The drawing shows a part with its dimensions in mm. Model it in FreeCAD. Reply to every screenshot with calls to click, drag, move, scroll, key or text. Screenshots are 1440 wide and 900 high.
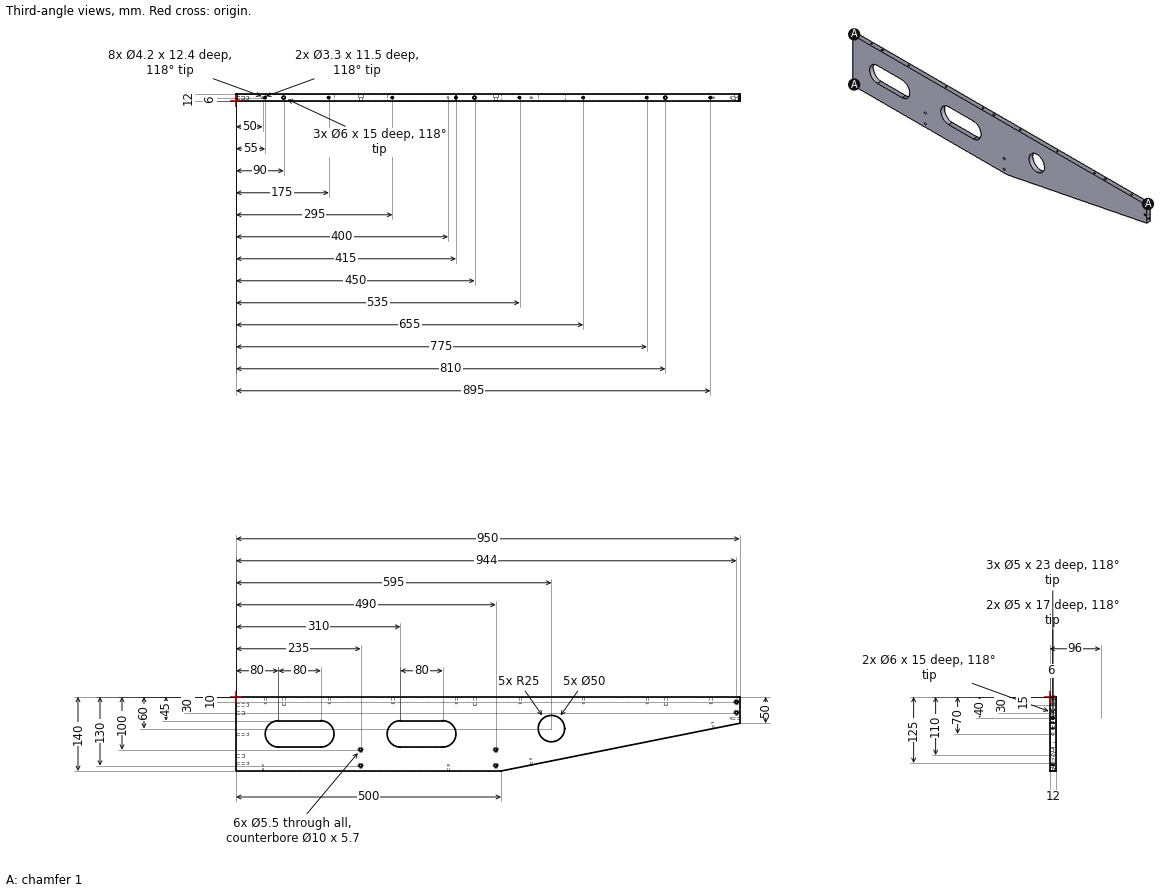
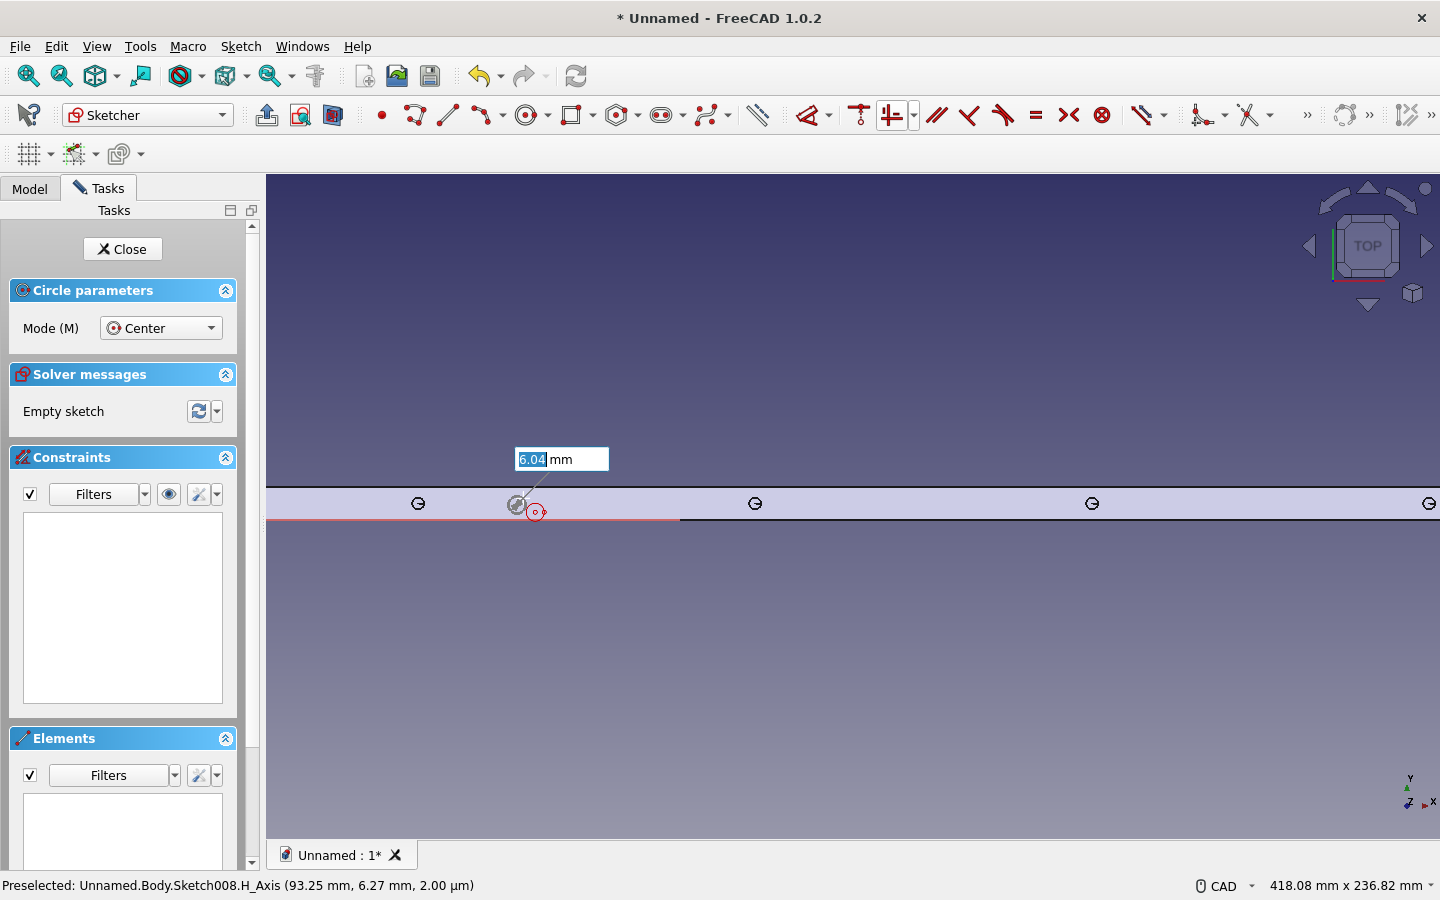
text(6)
key(Return)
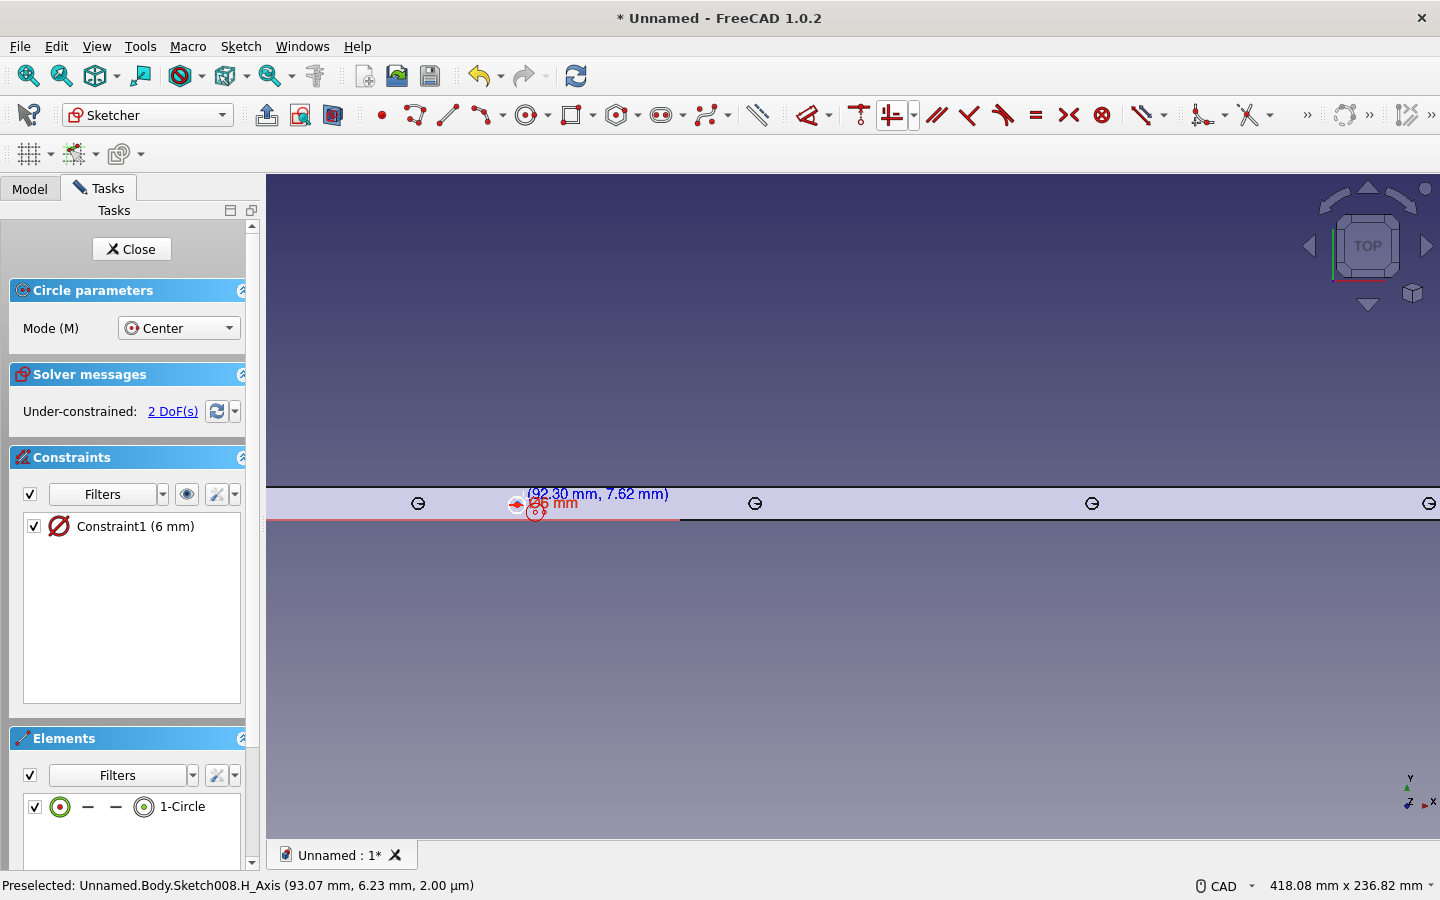
scroll(517, 506, down, 6)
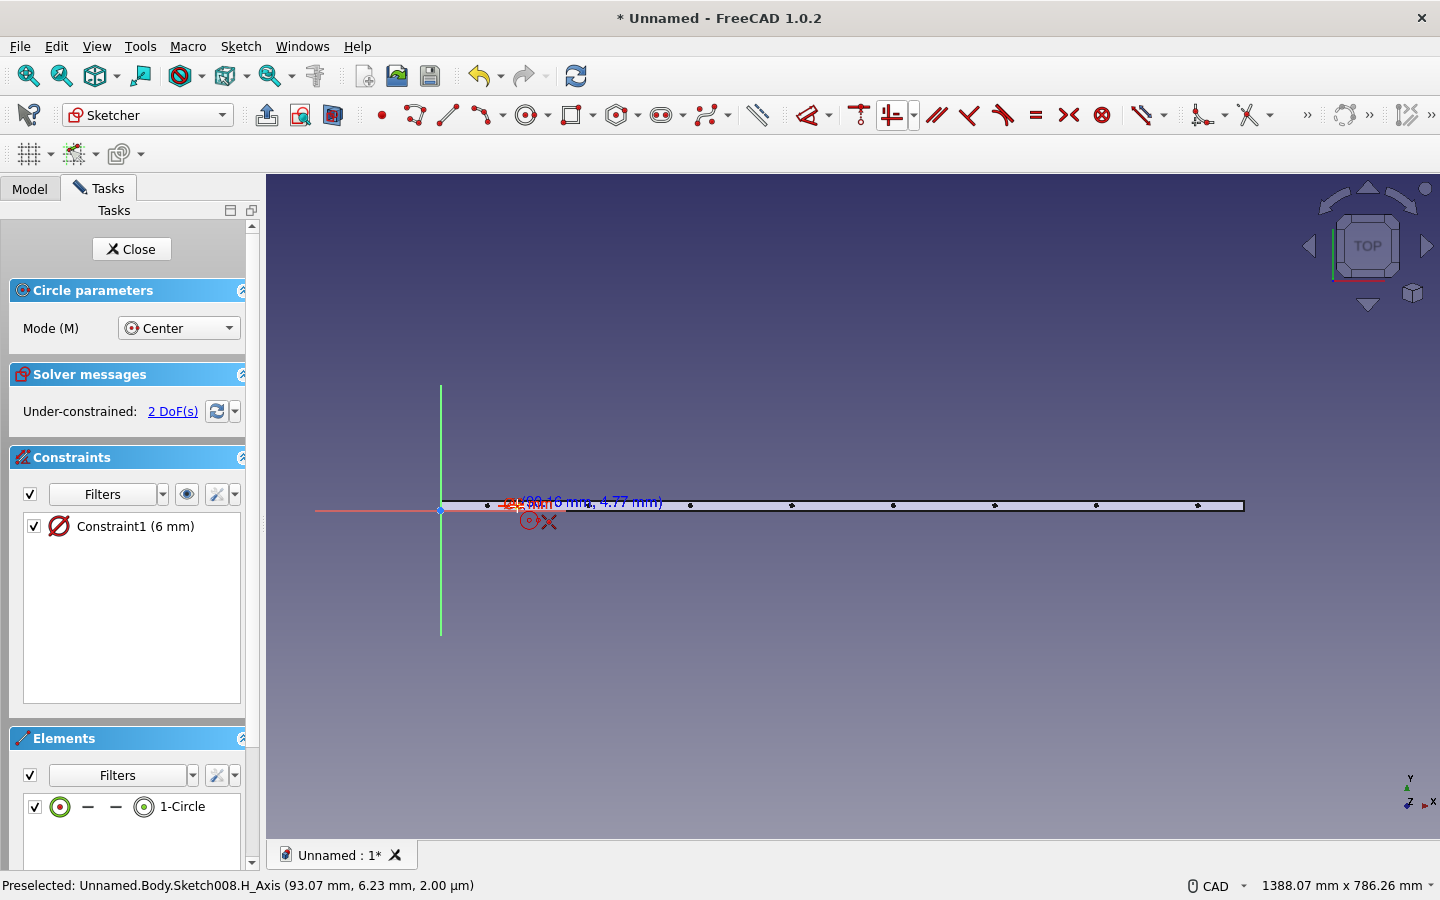
scroll(821, 506, up, 11)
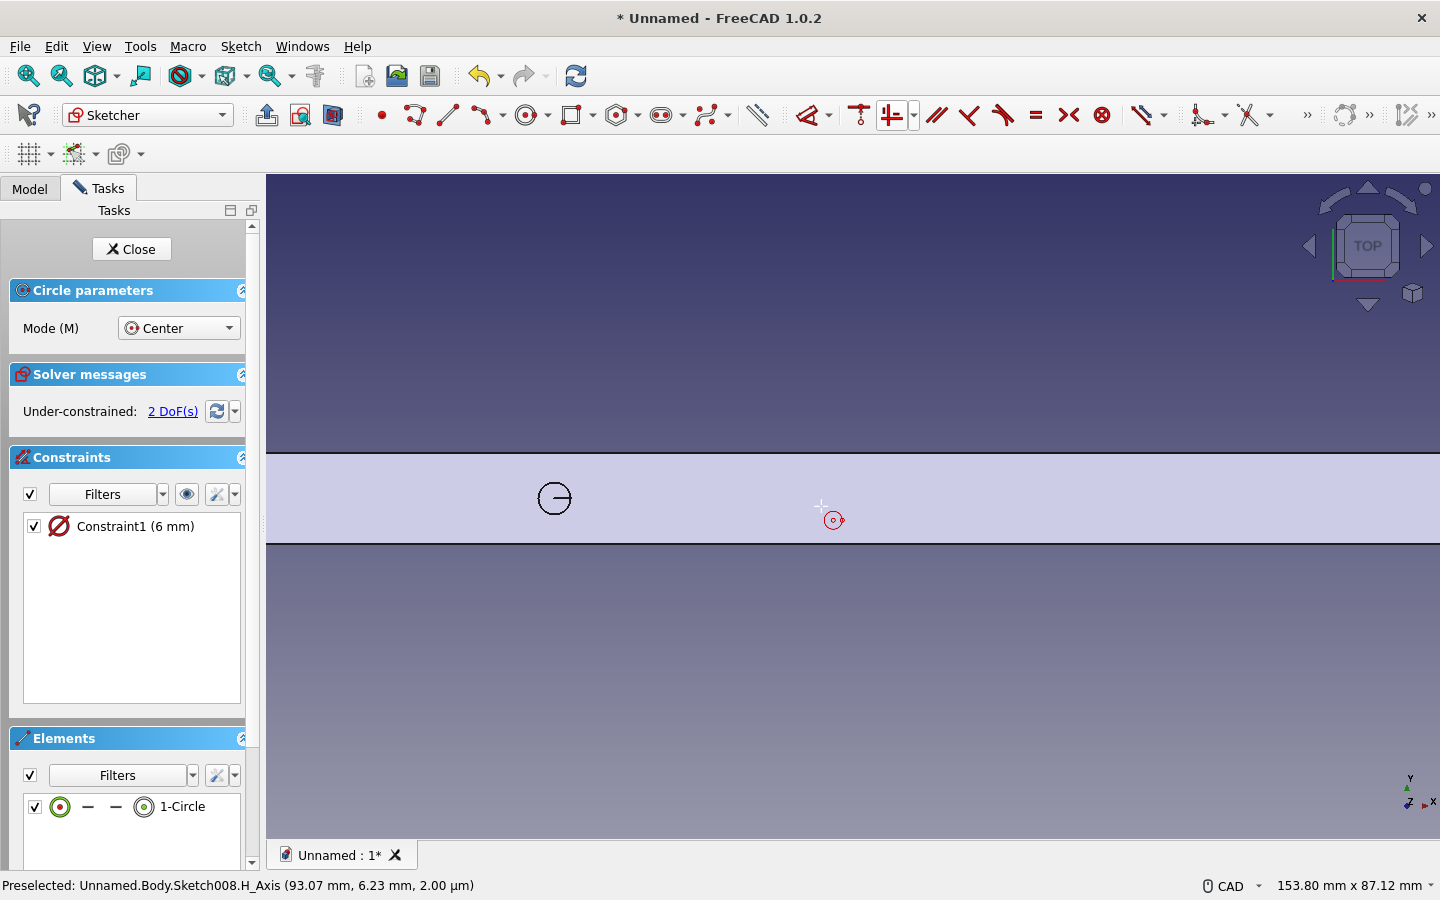
scroll(821, 506, down, 11)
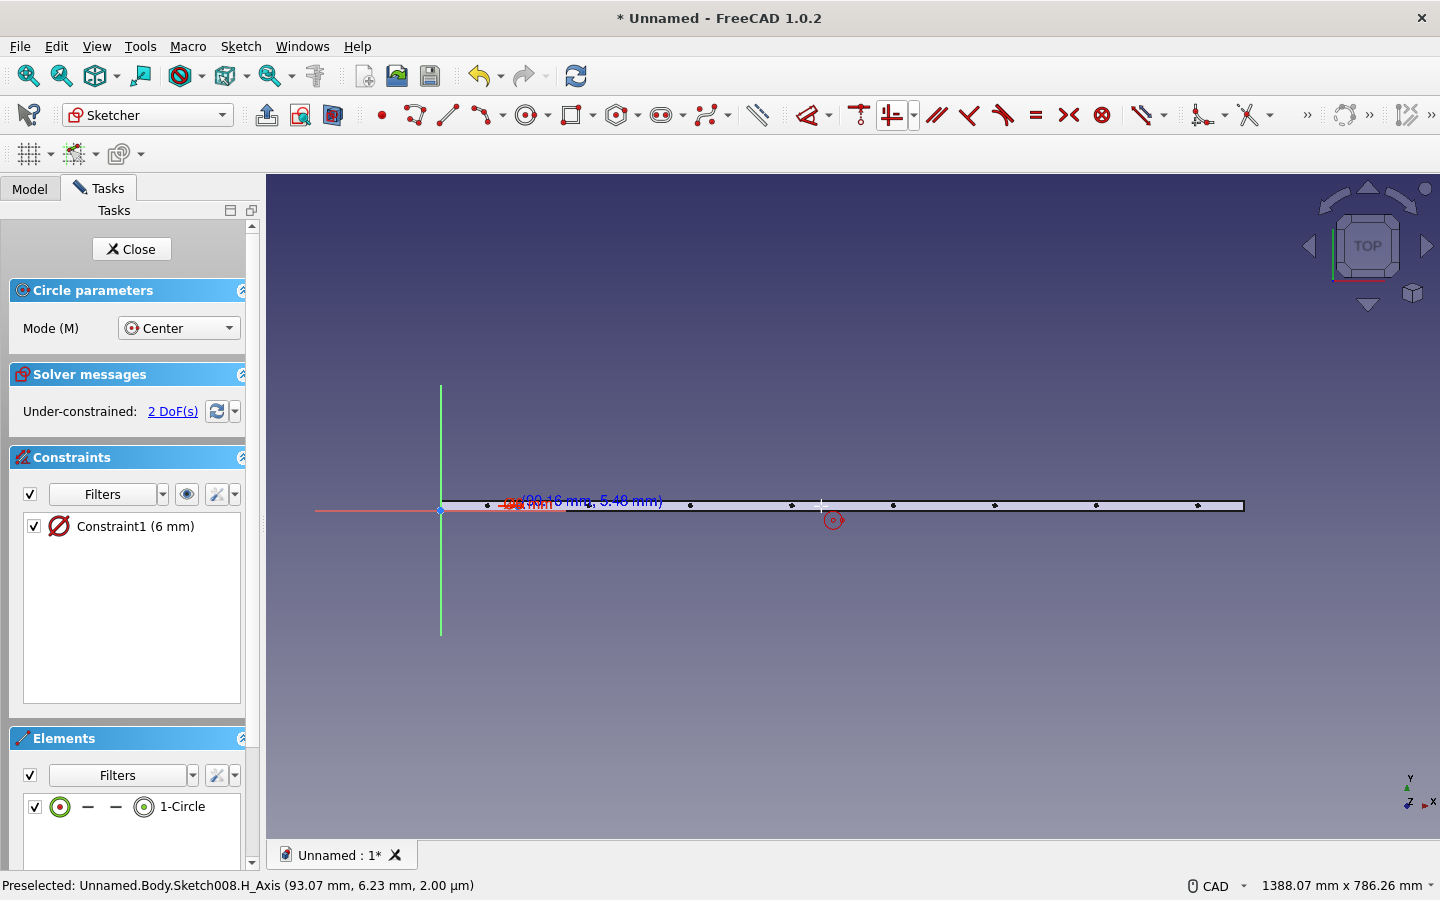
scroll(821, 506, up, 6)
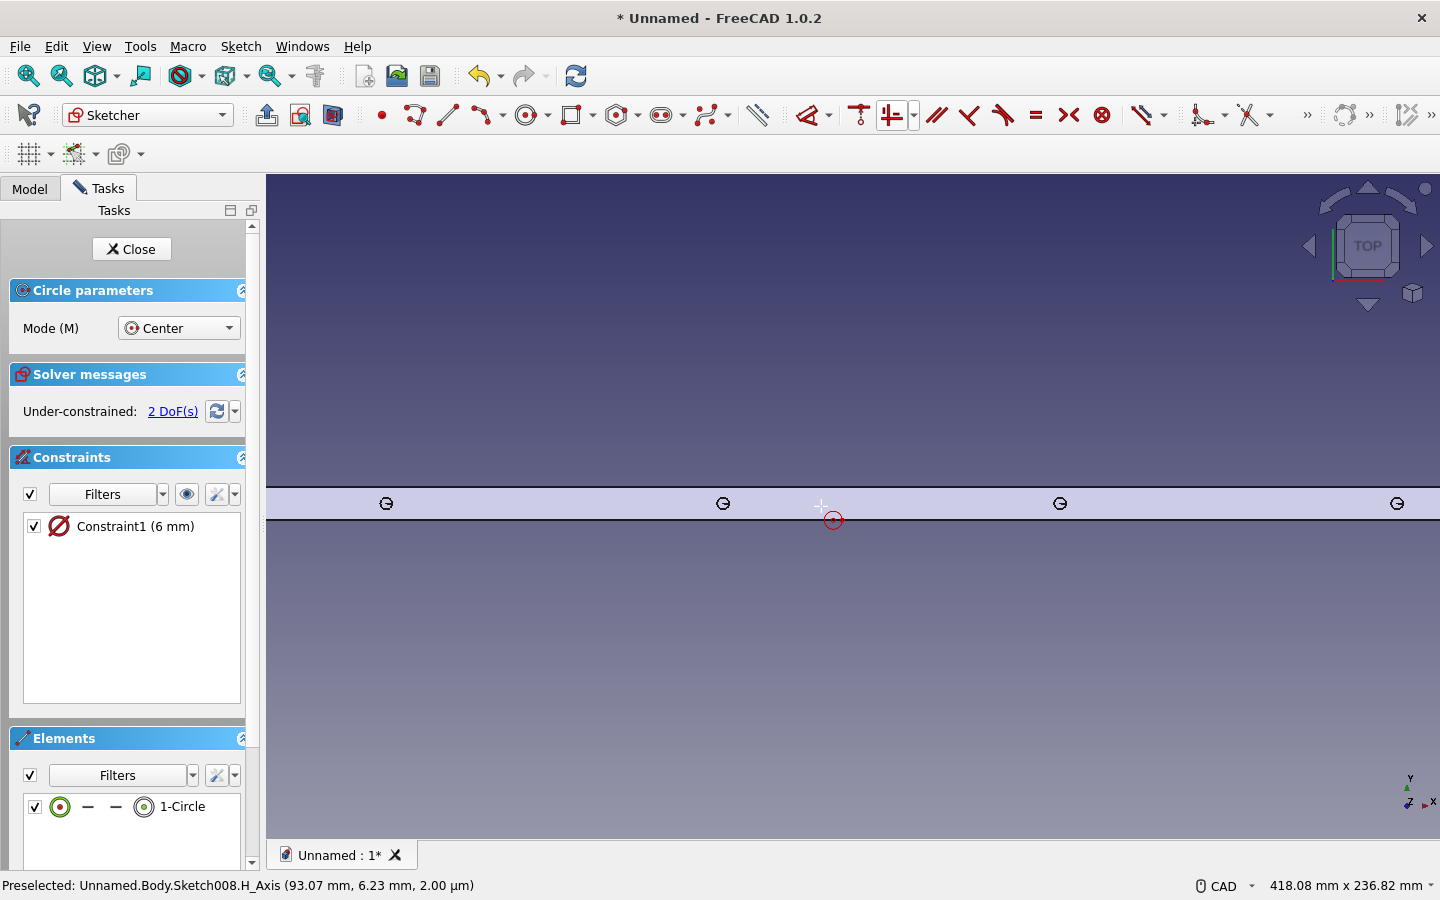
click(822, 504)
move(827, 498)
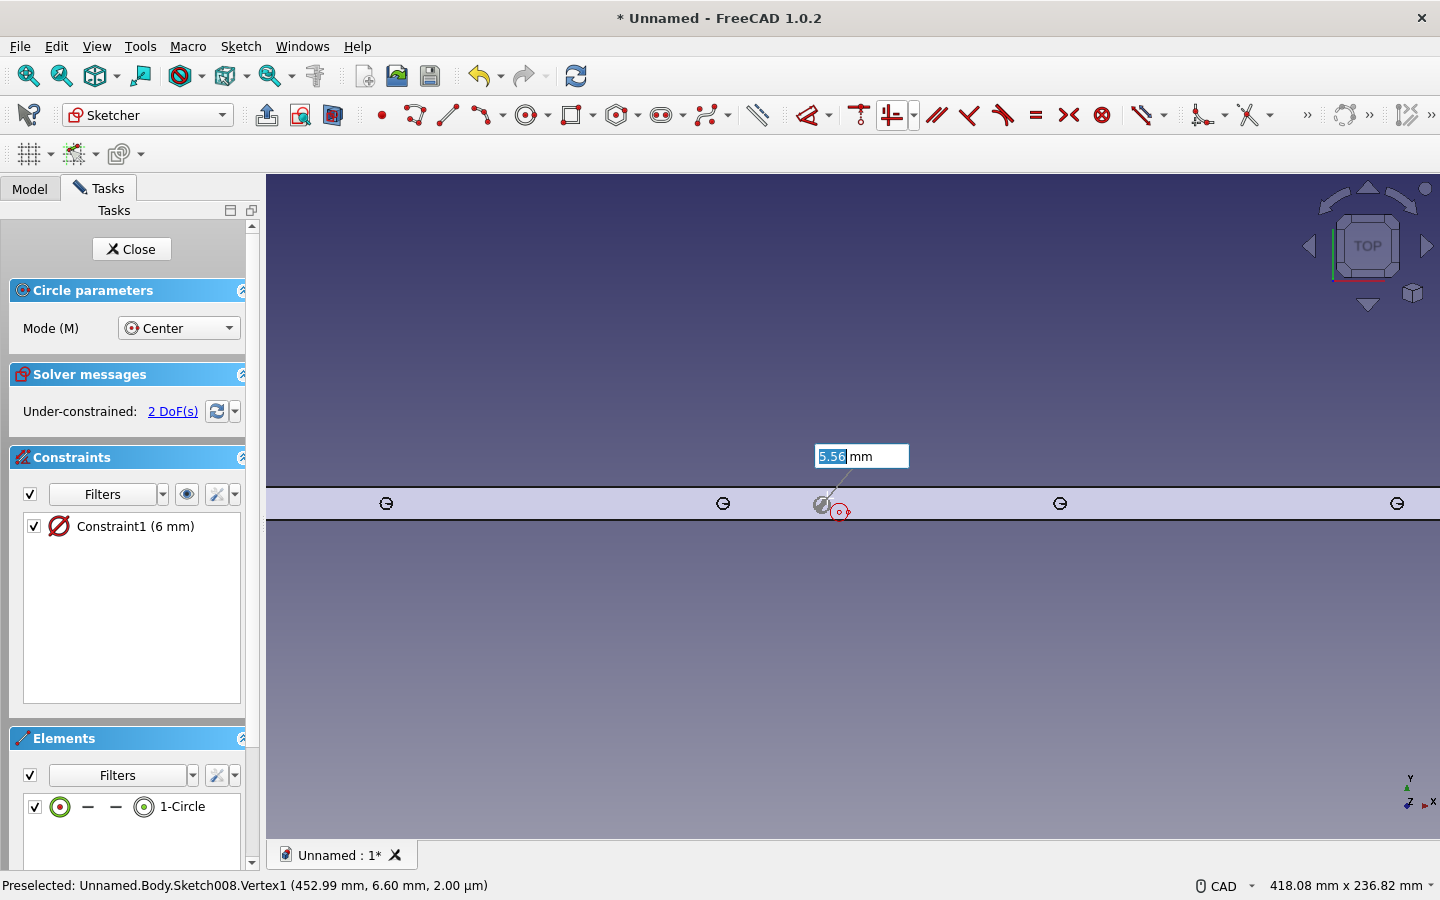
text(6)
key(Return)